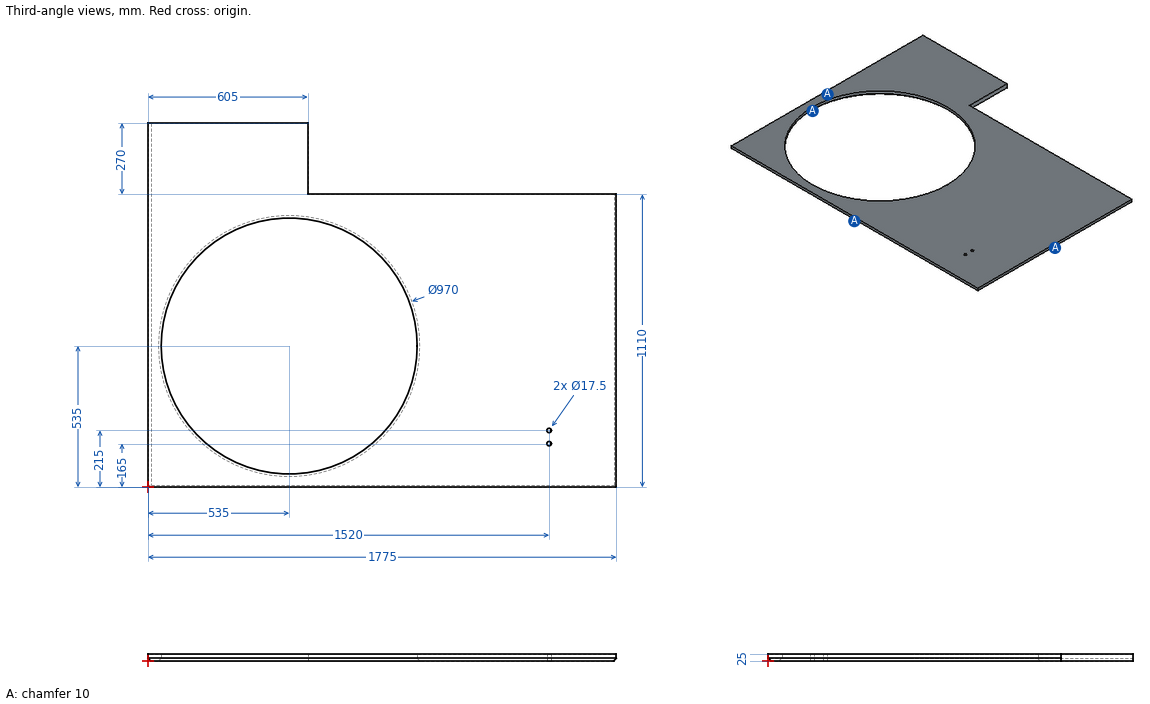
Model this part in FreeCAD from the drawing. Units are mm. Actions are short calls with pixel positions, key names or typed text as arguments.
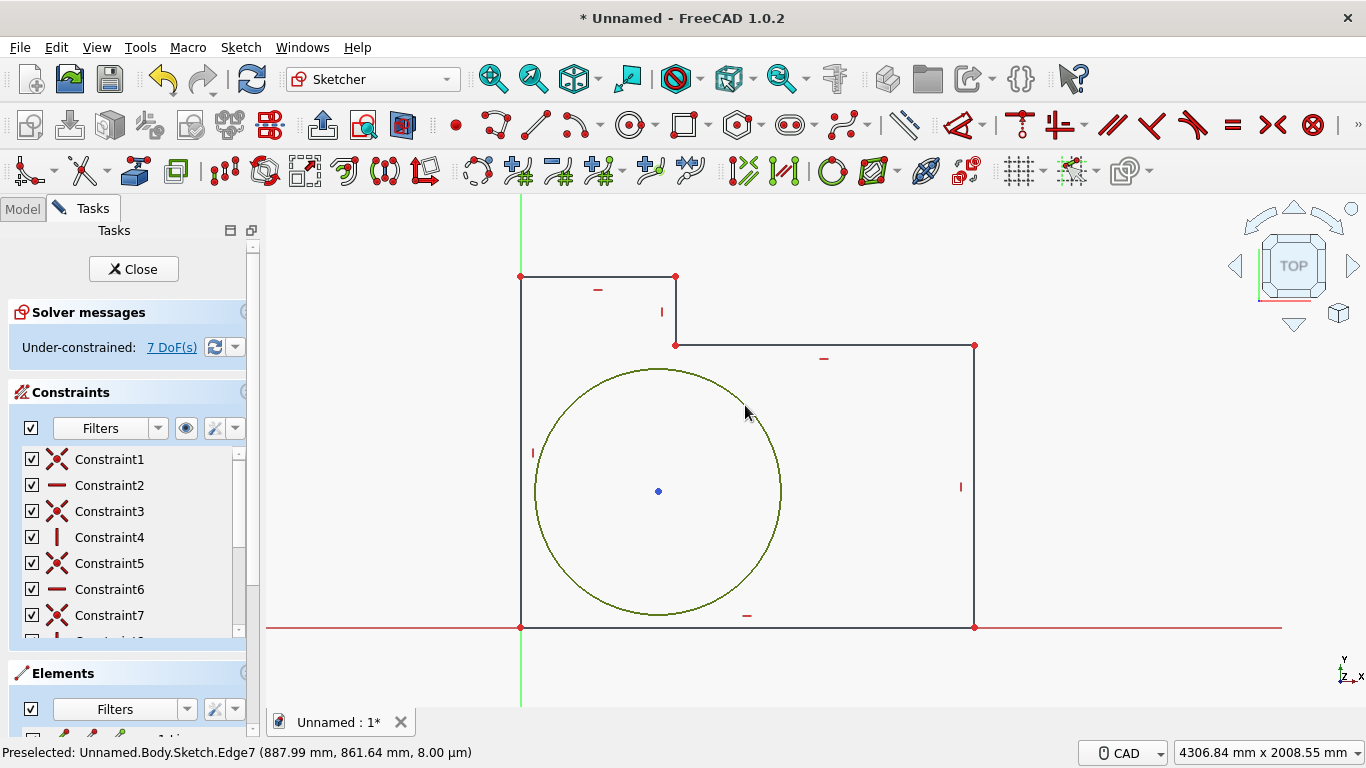
key(k)
key(o)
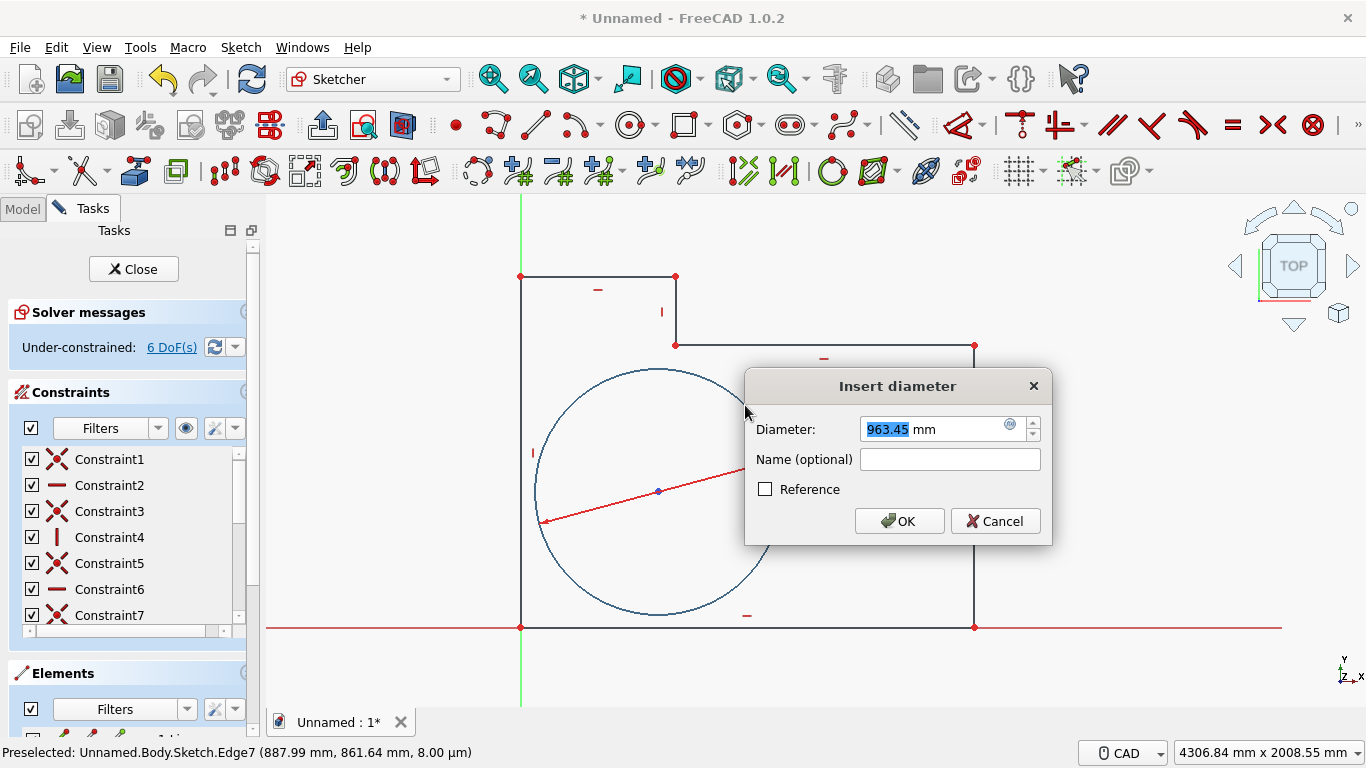
text(970)
key(Return)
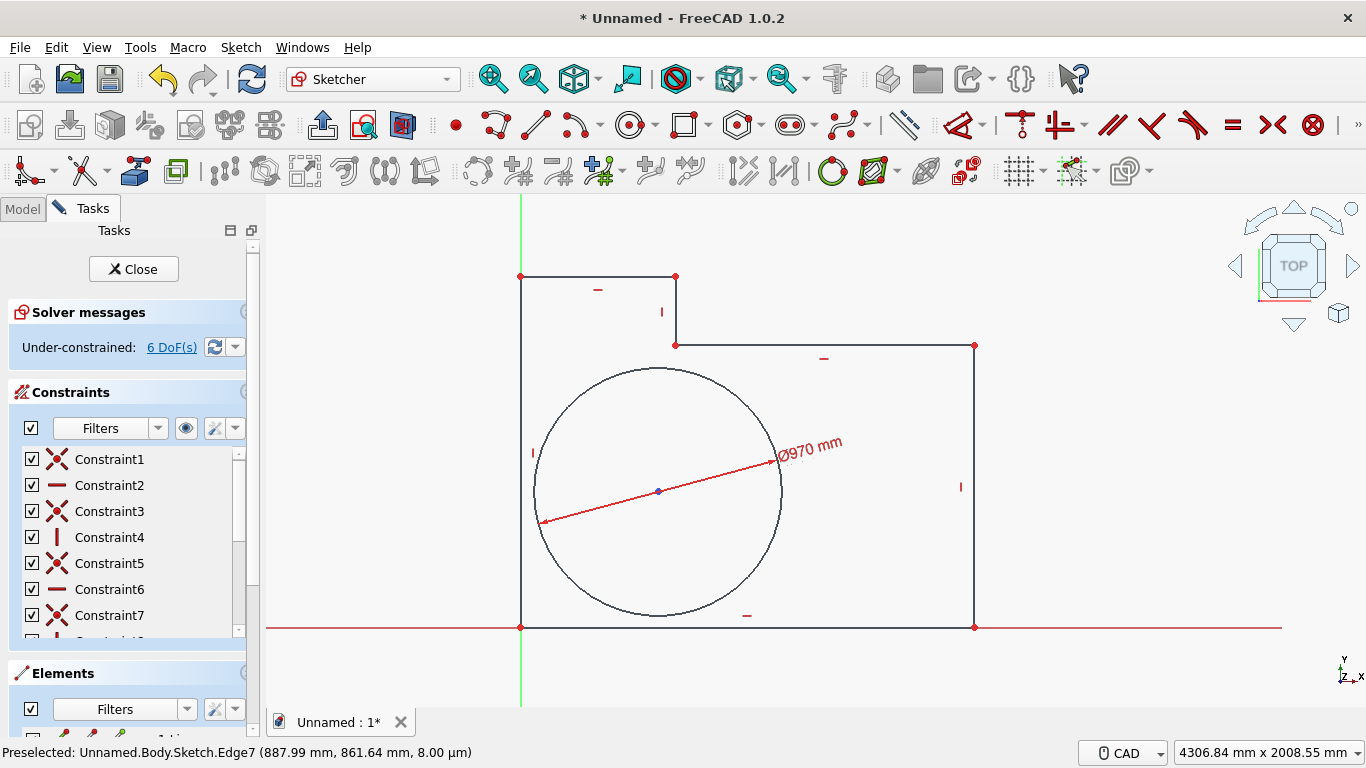
click(676, 325)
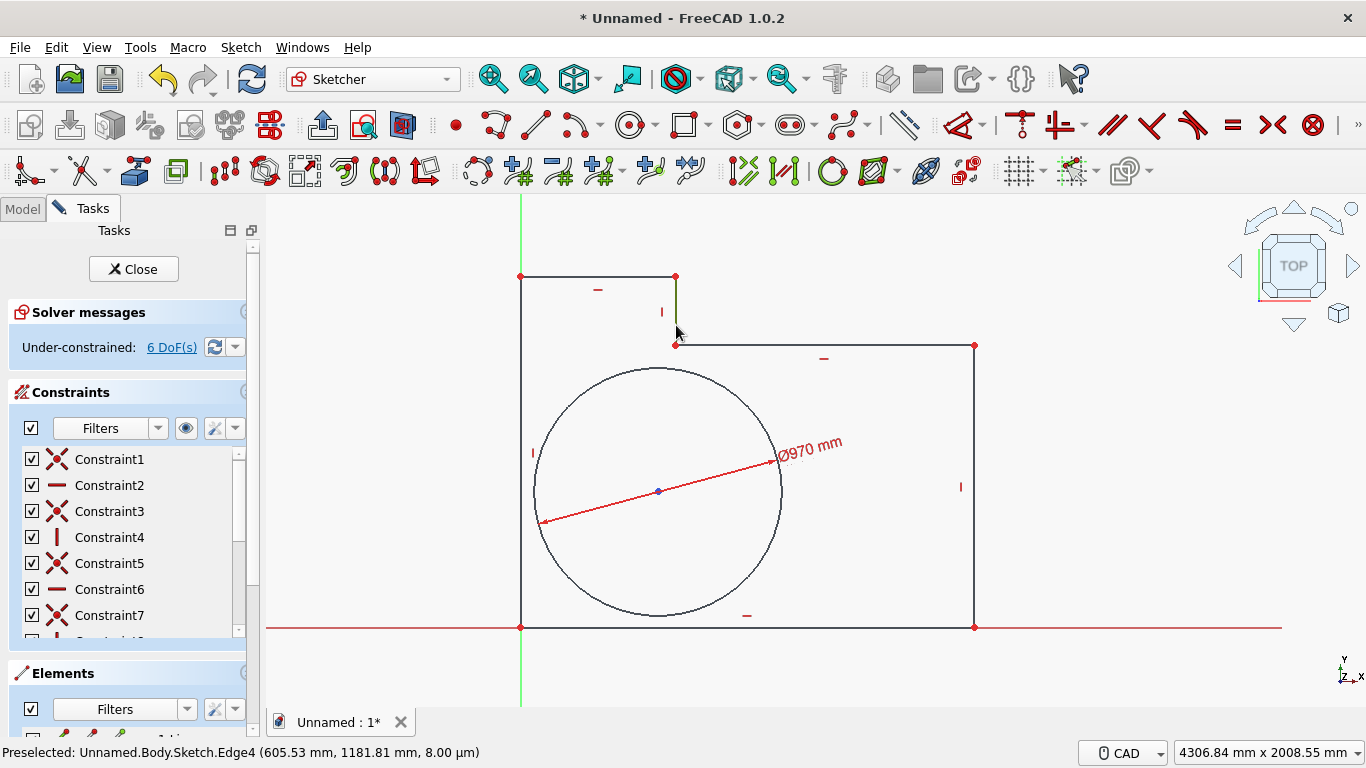
click(984, 126)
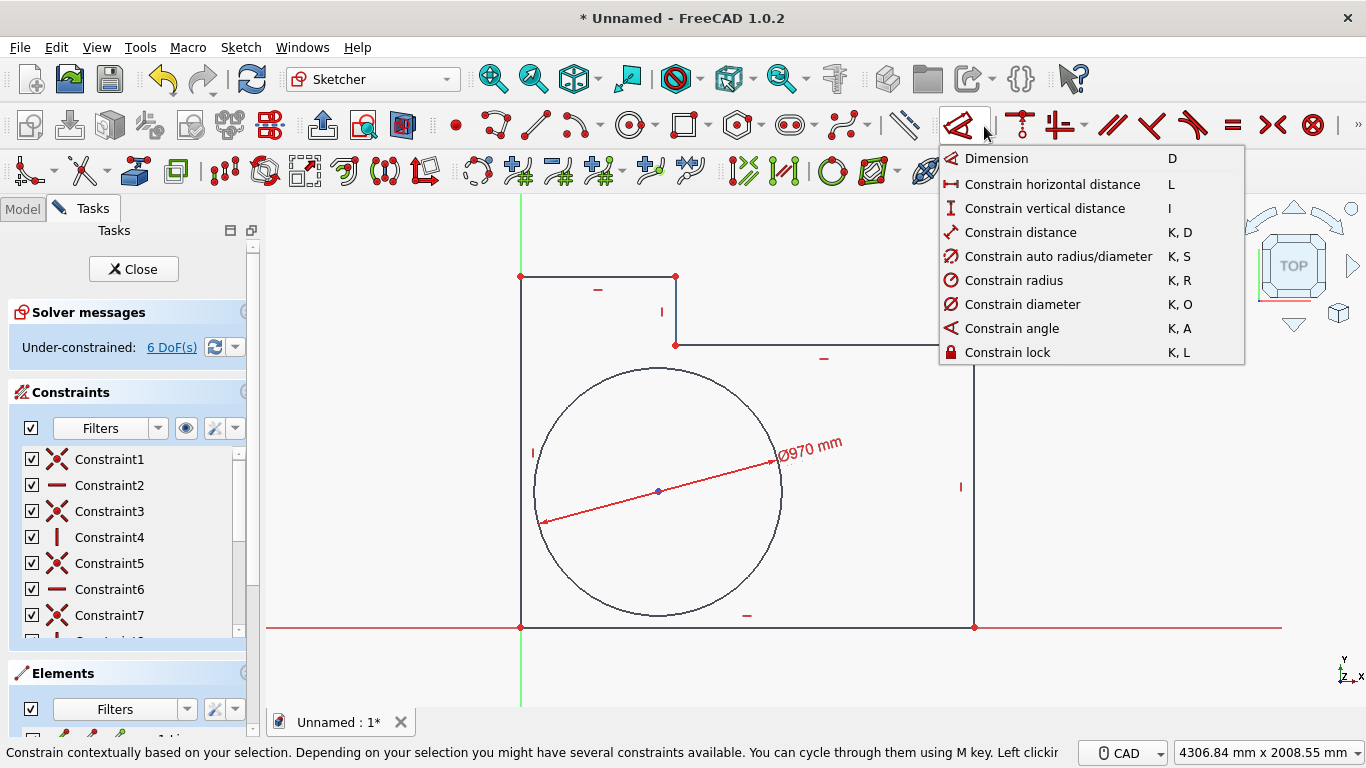
click(1092, 208)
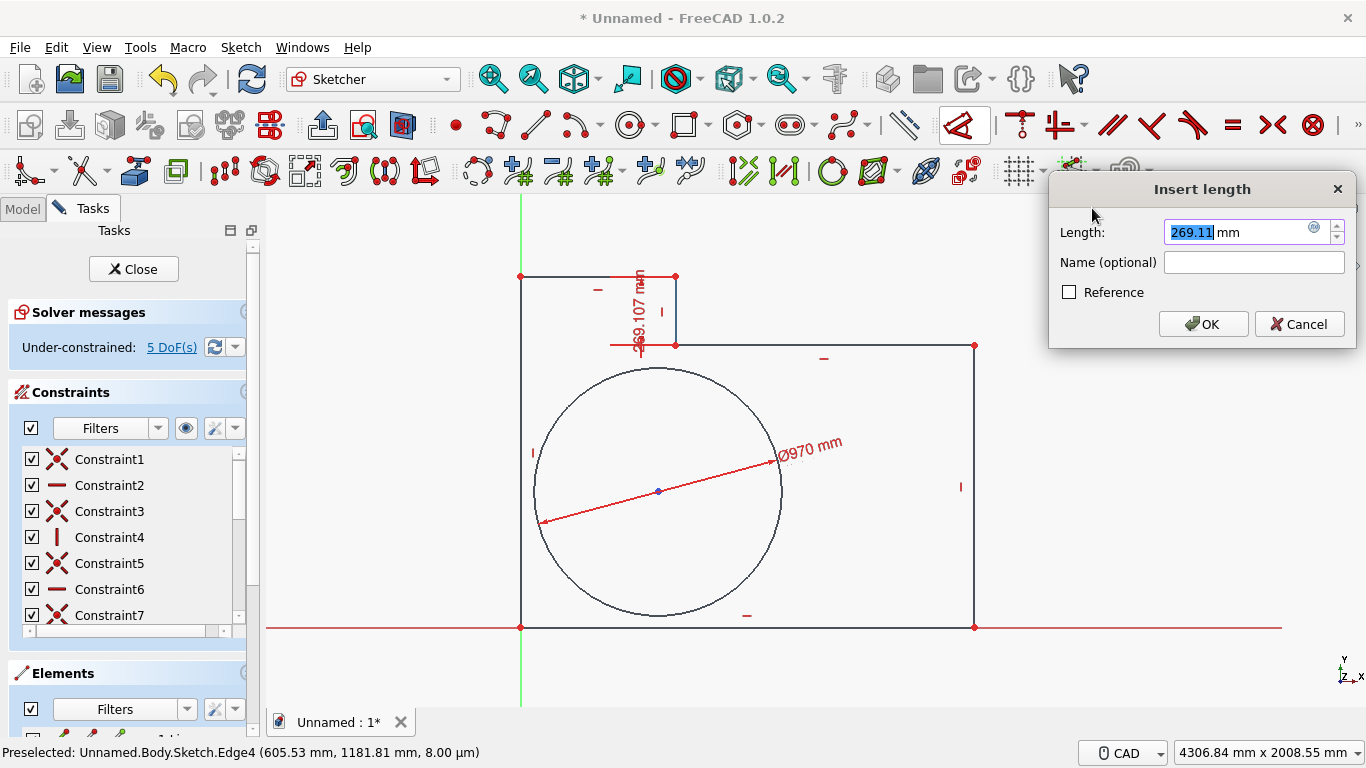
text(270)
key(Return)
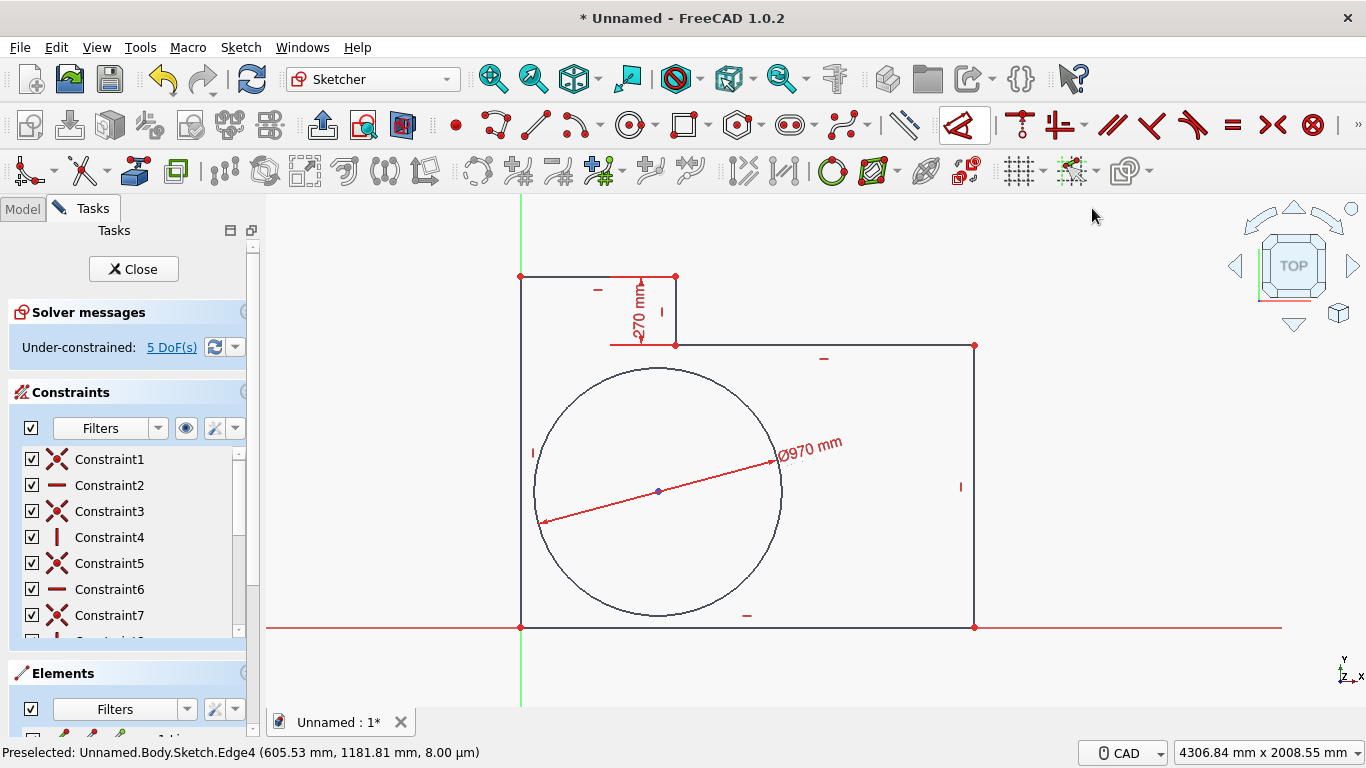
click(629, 277)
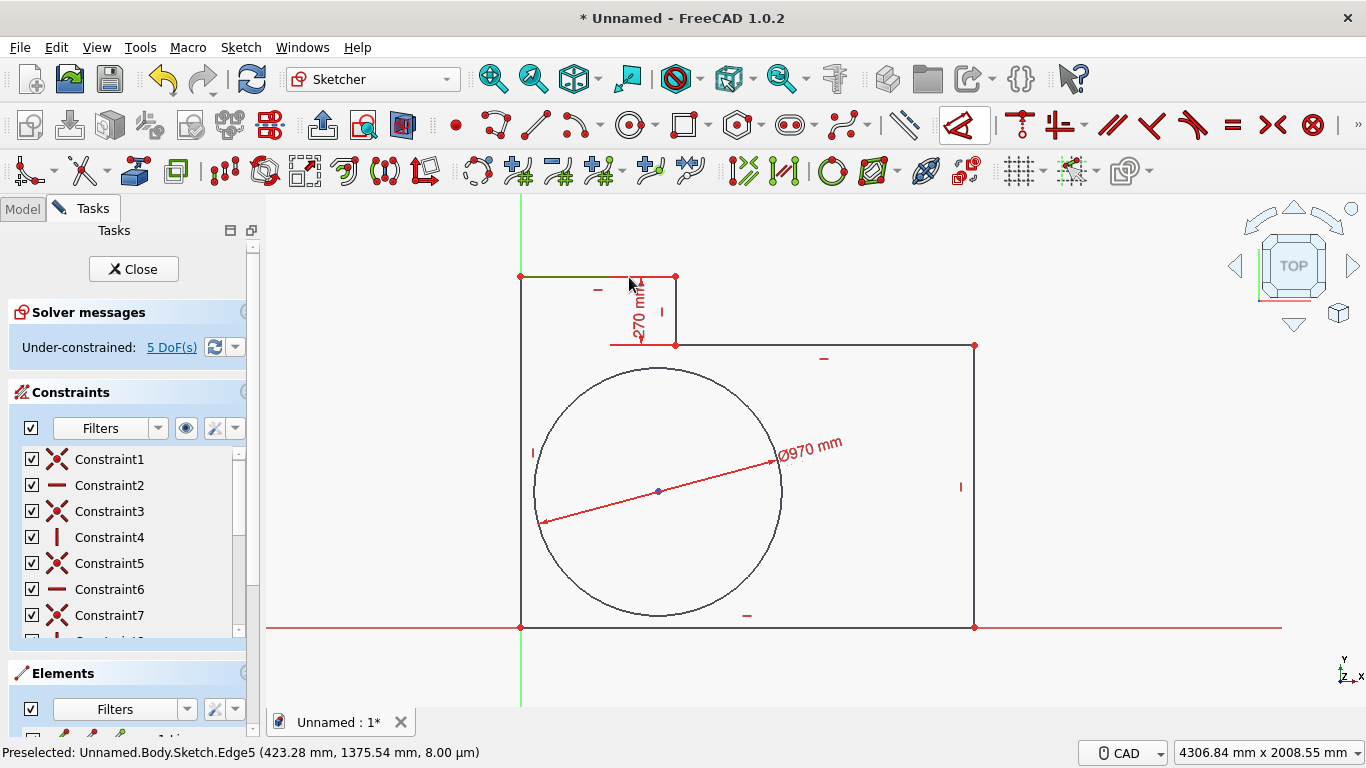
click(984, 126)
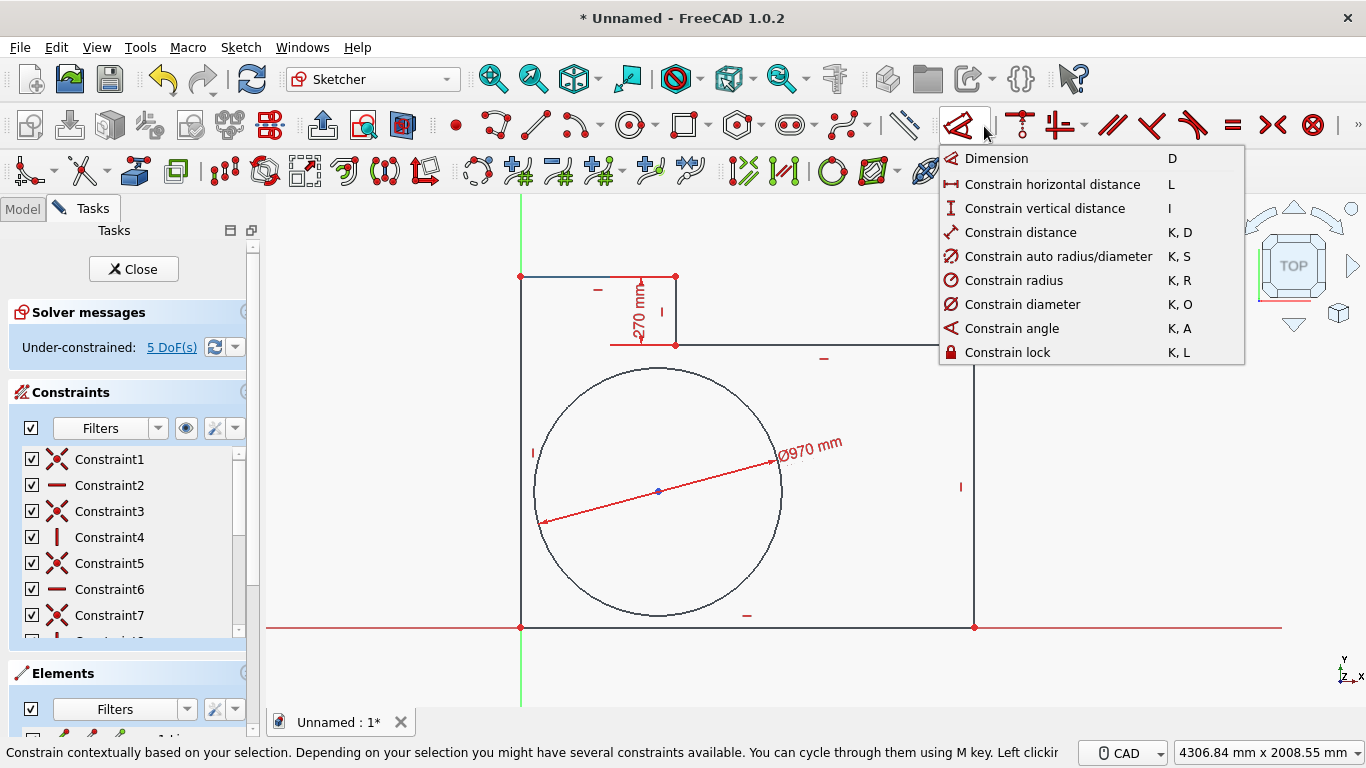
click(1092, 184)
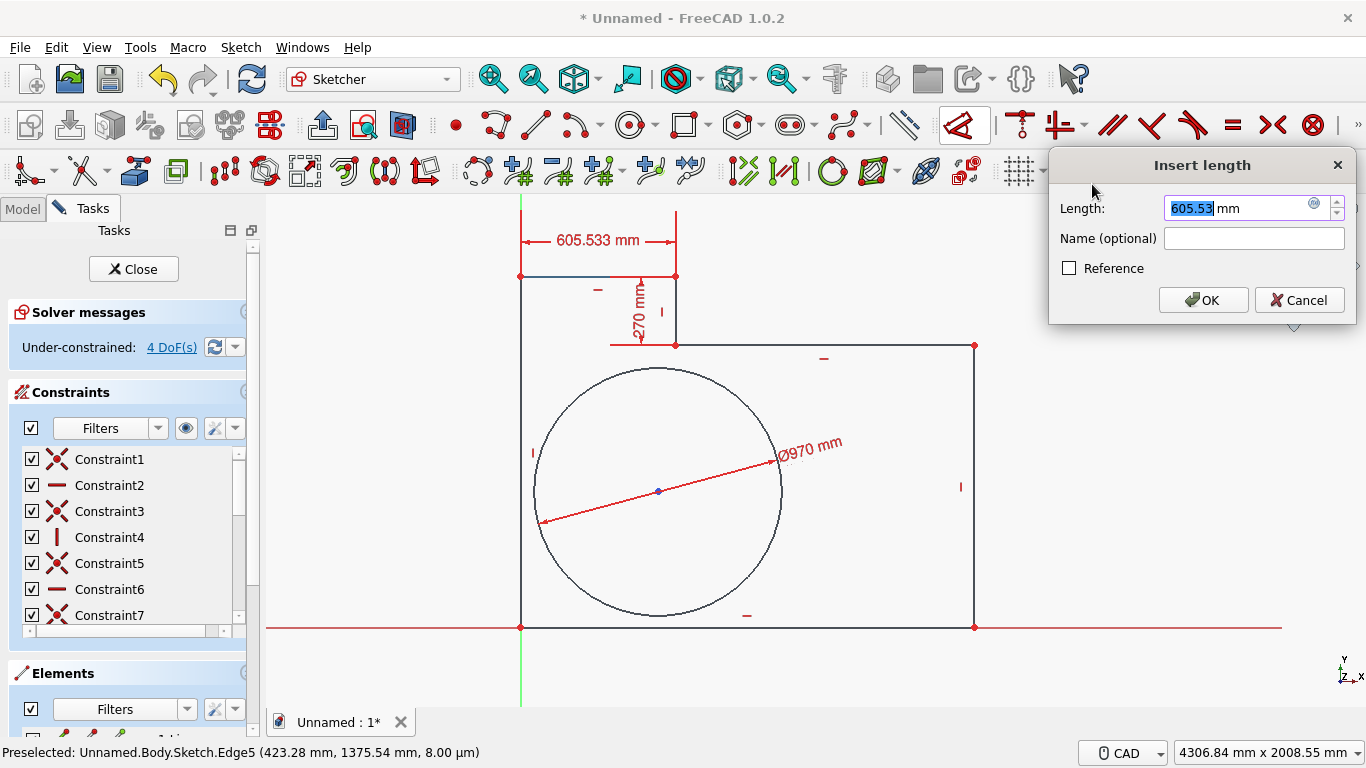
text(605)
key(Return)